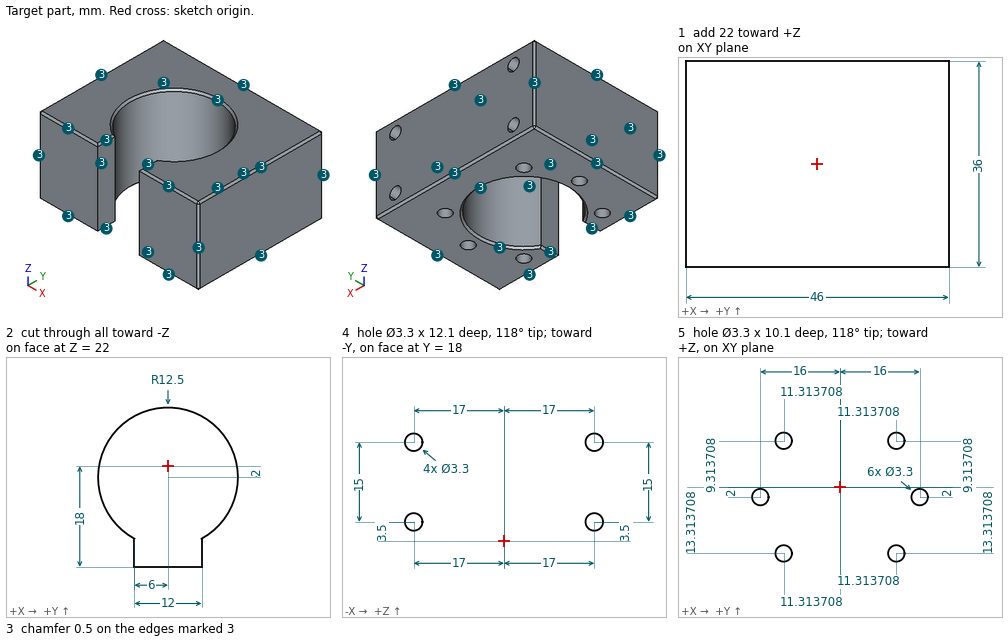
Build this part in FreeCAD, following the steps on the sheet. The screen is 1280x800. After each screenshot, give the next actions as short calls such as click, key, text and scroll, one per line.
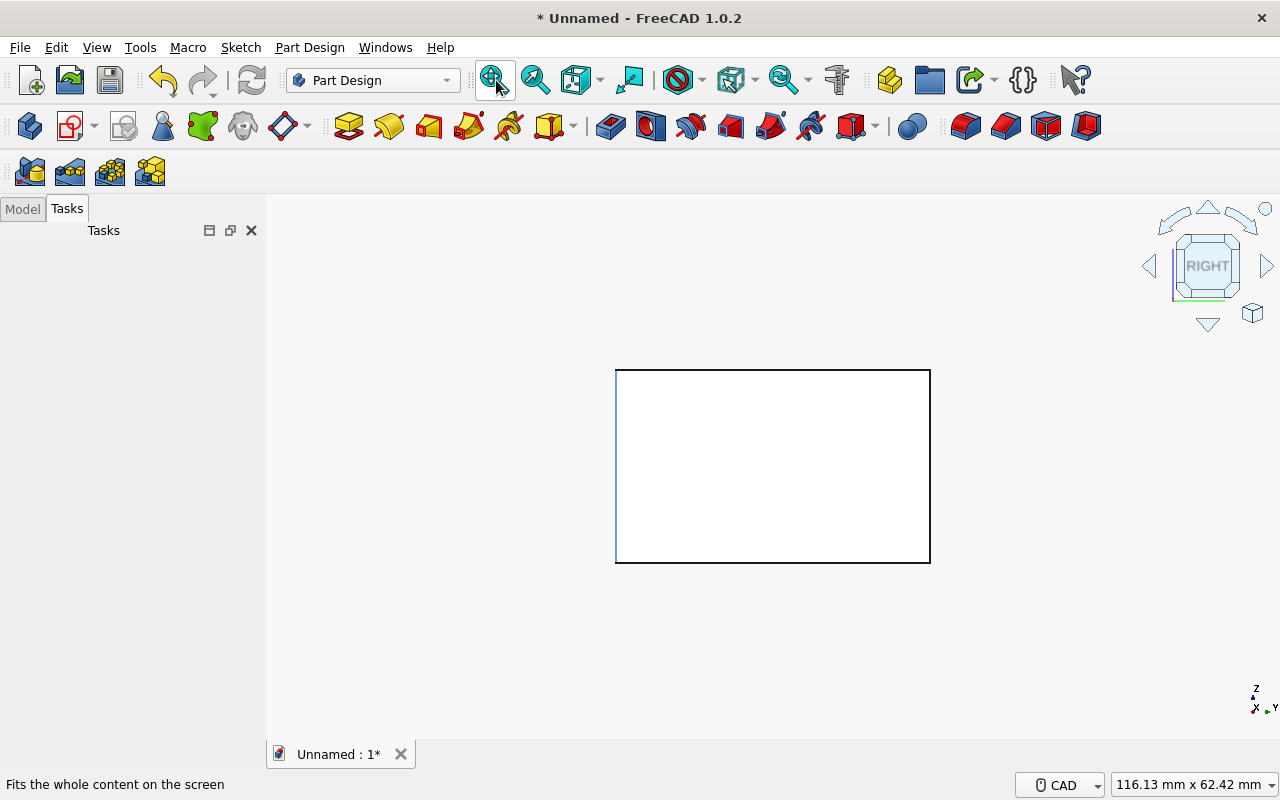
click(930, 465, ctrl)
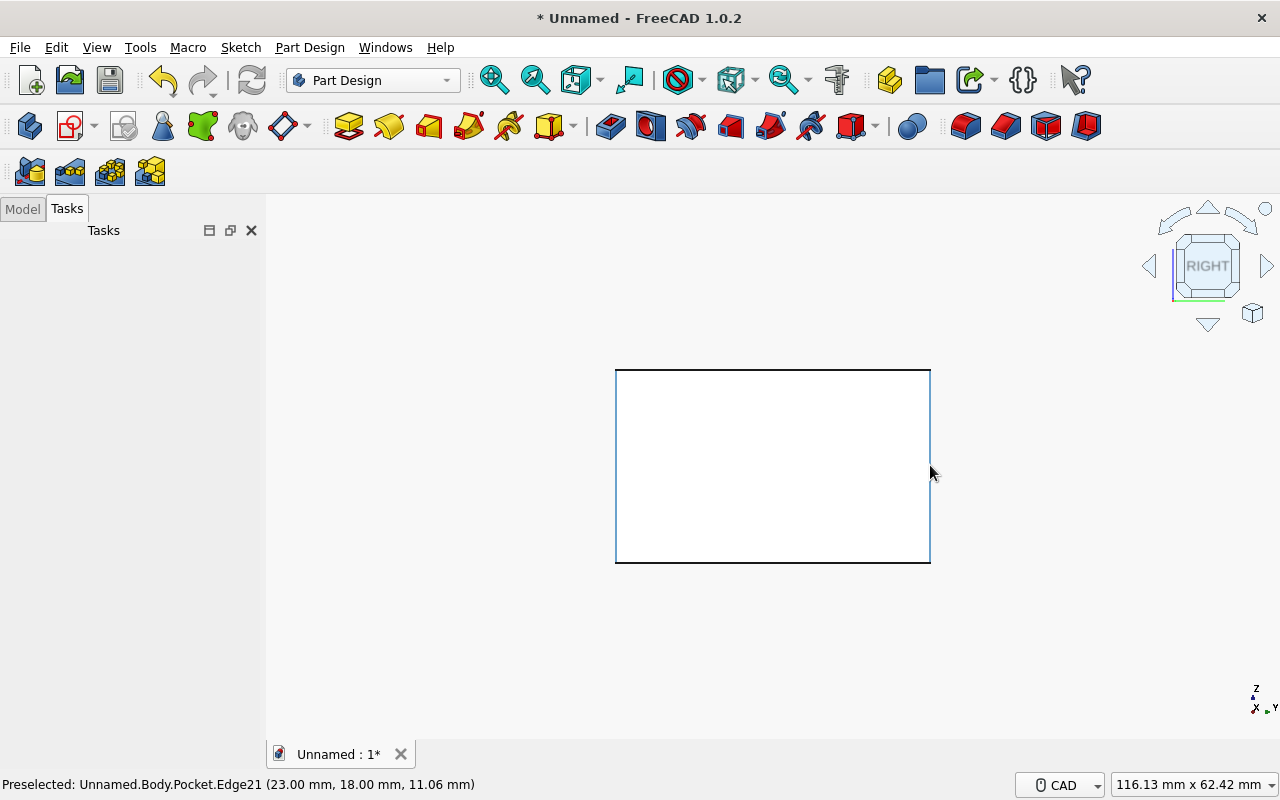
key(5)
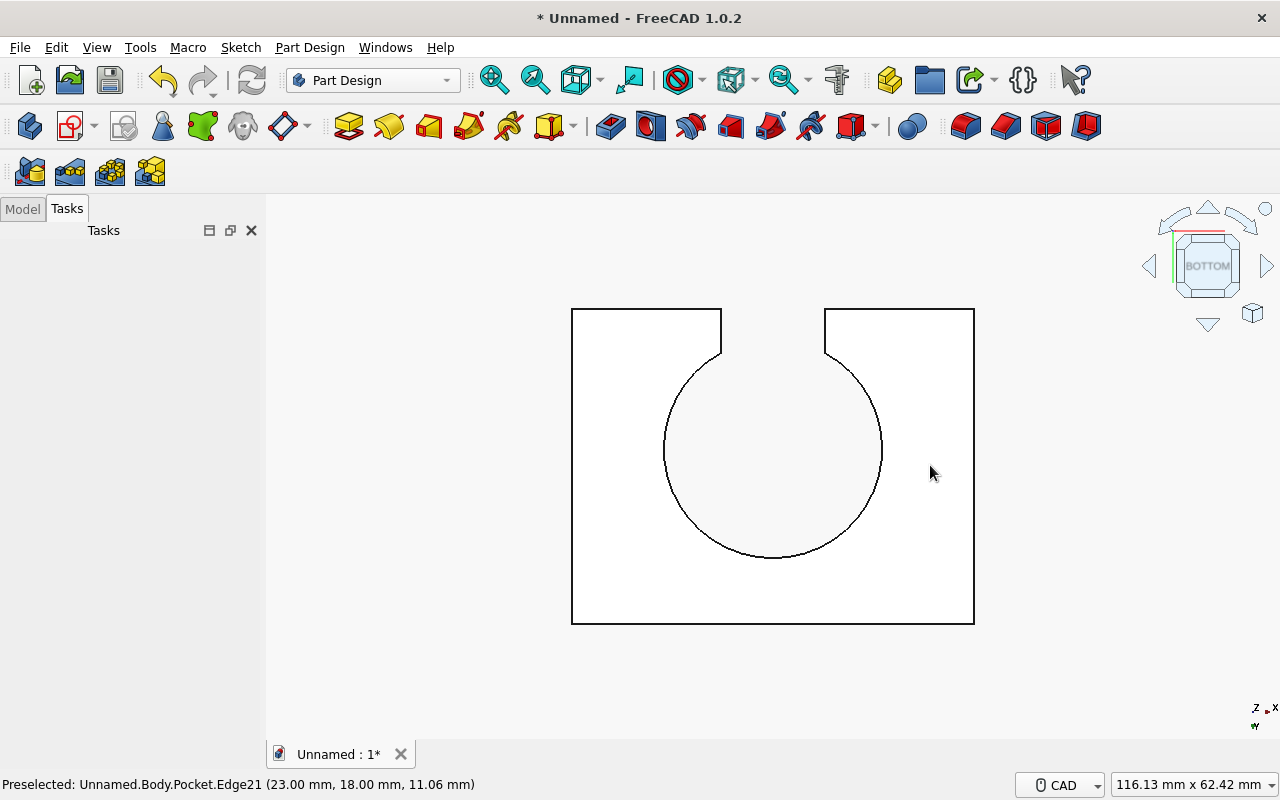
click(888, 555, ctrl)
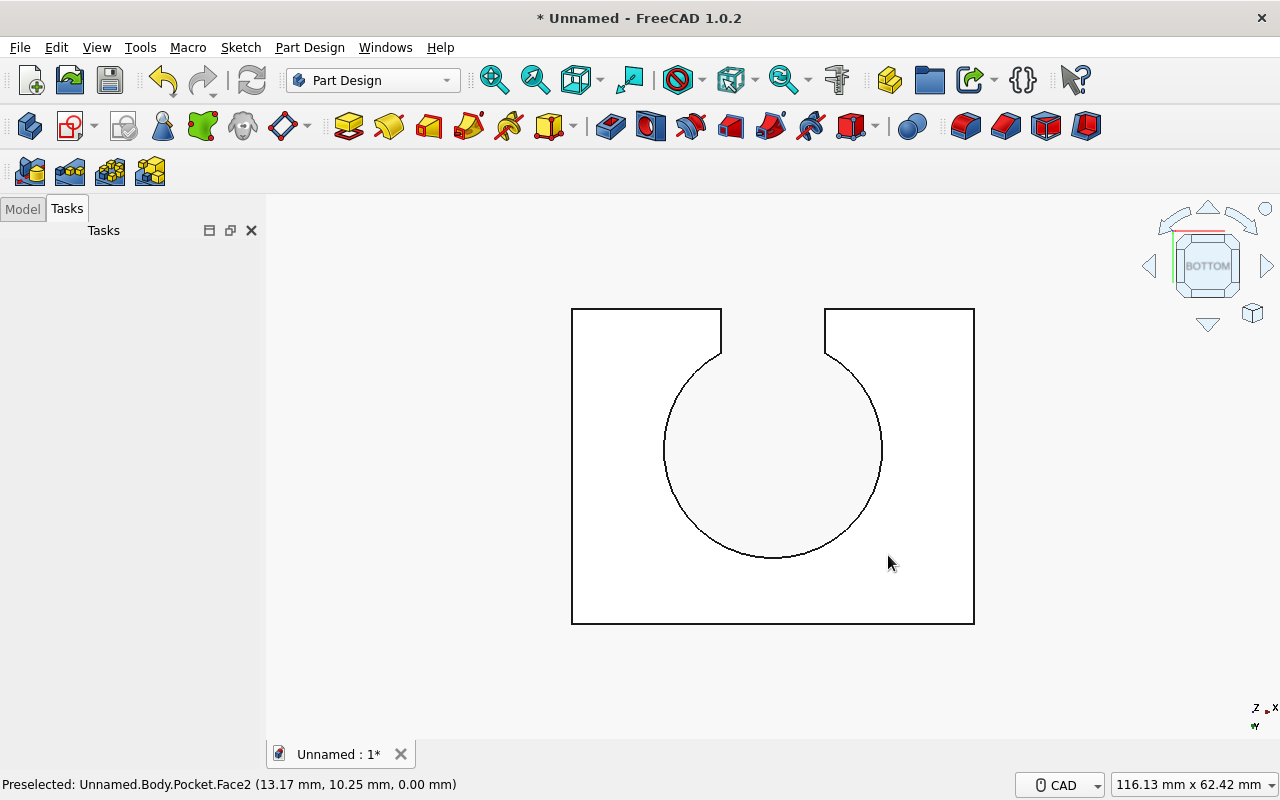
key(4)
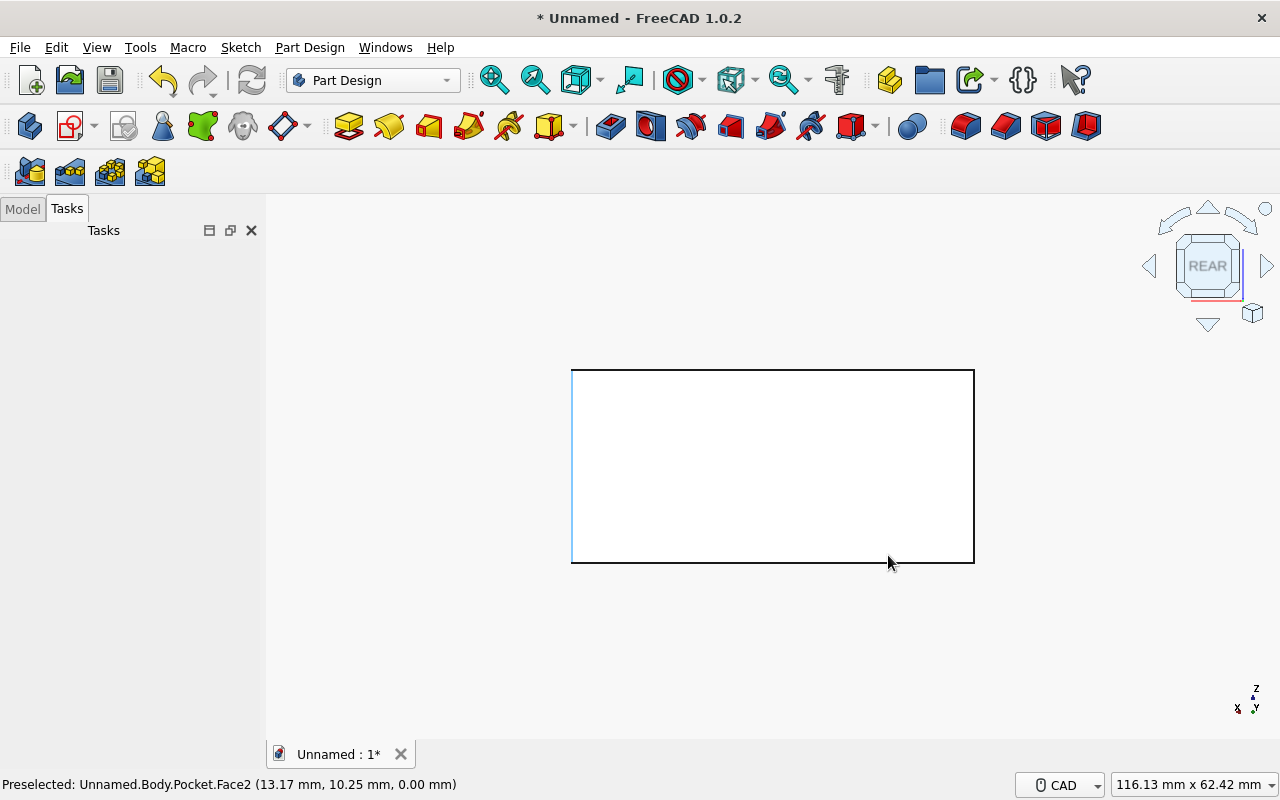
click(496, 80)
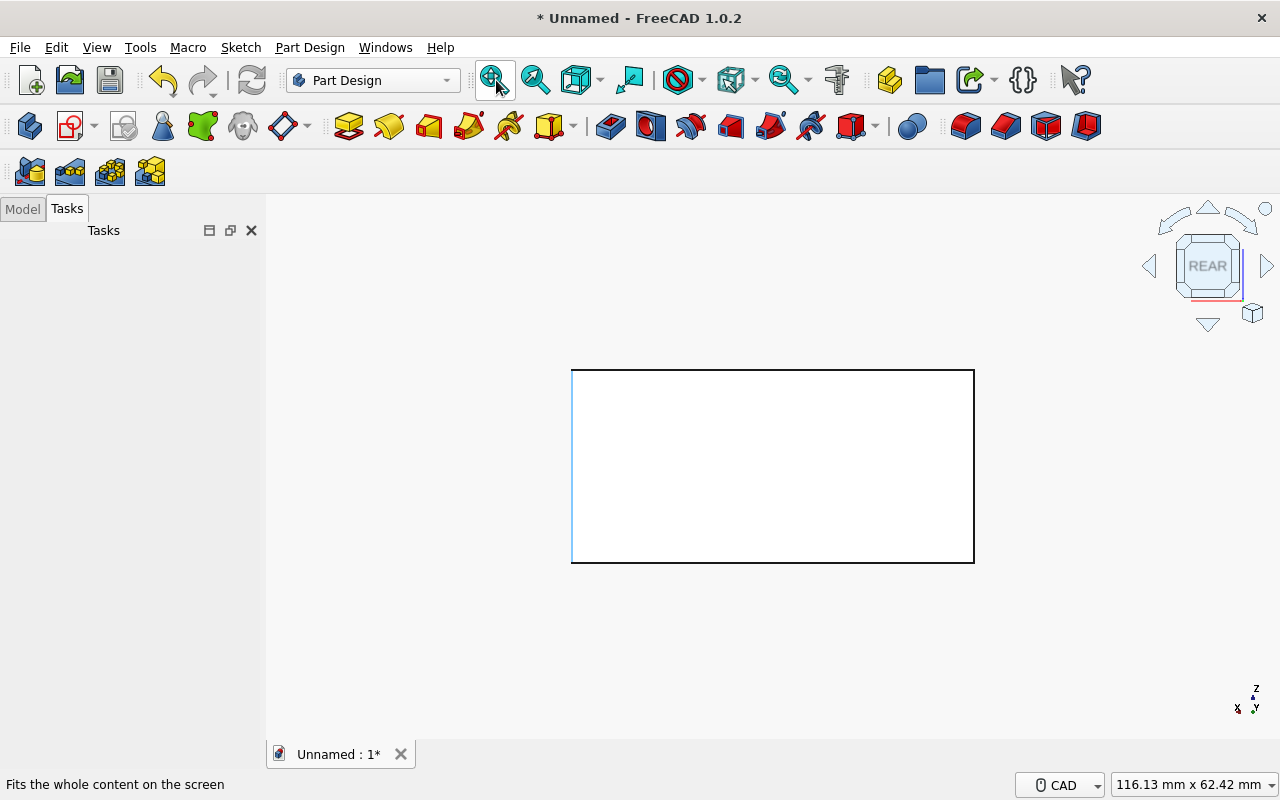
click(974, 466, ctrl)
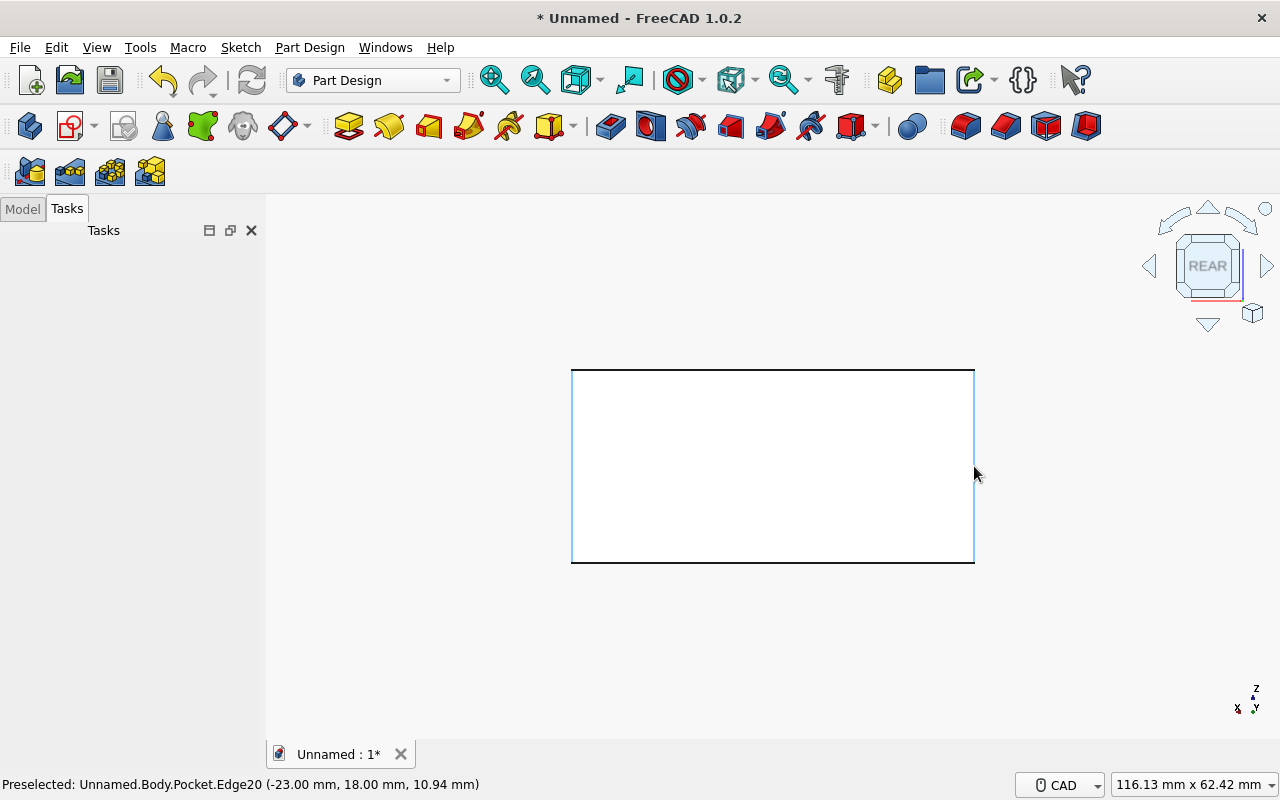
click(1006, 126)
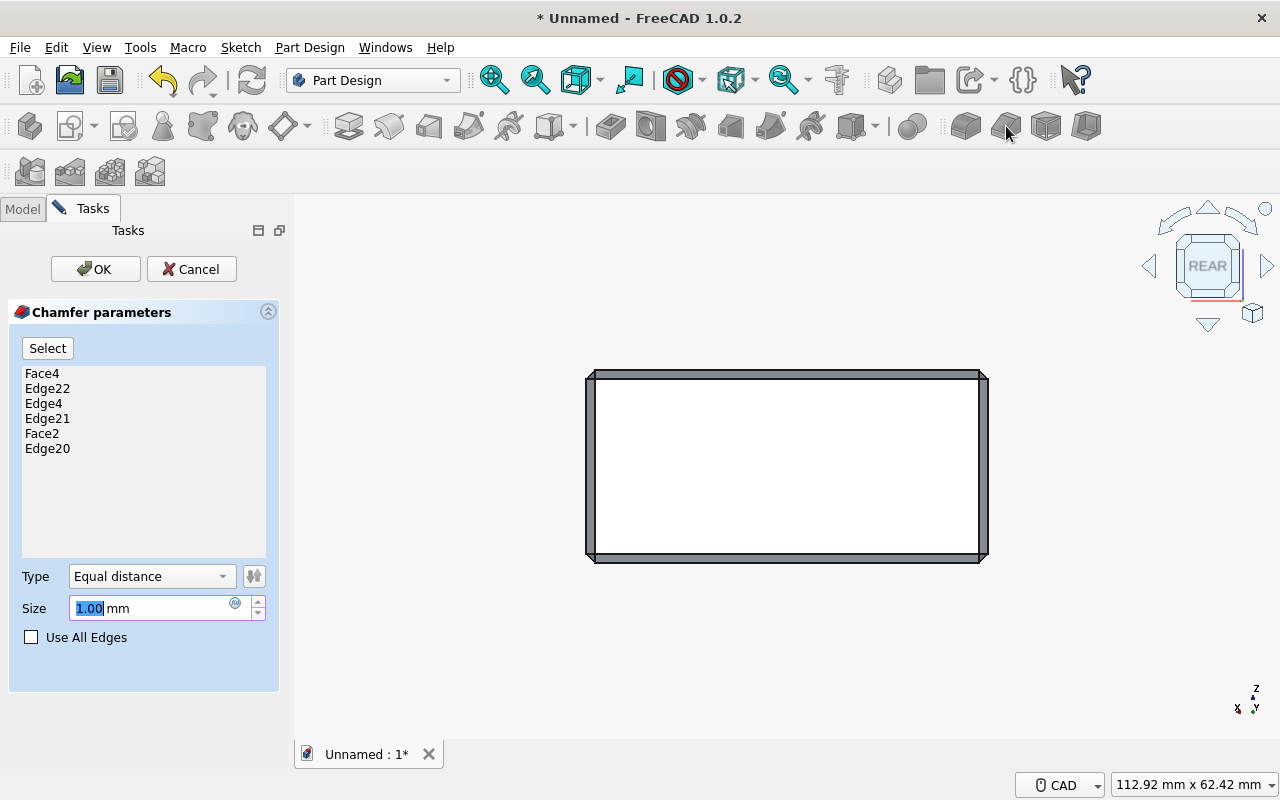
text(0.5)
key(Tab)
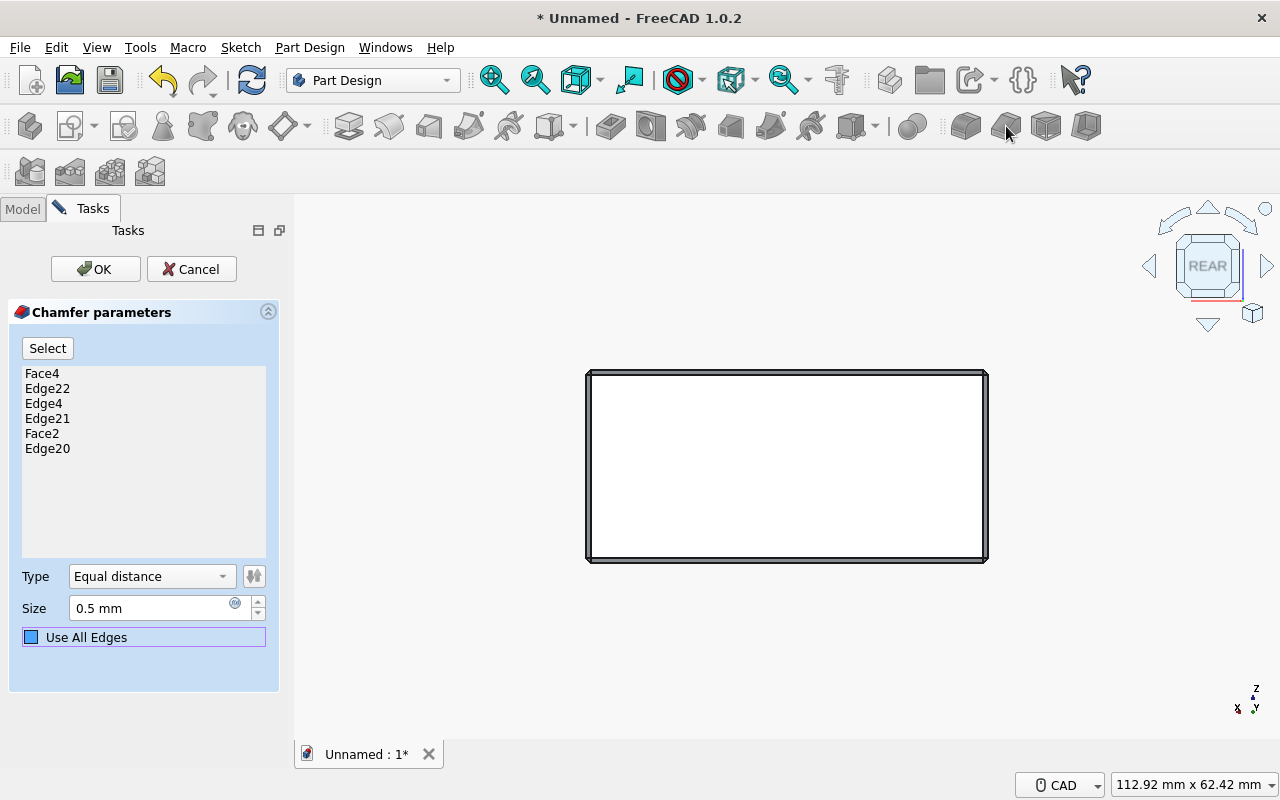
click(96, 269)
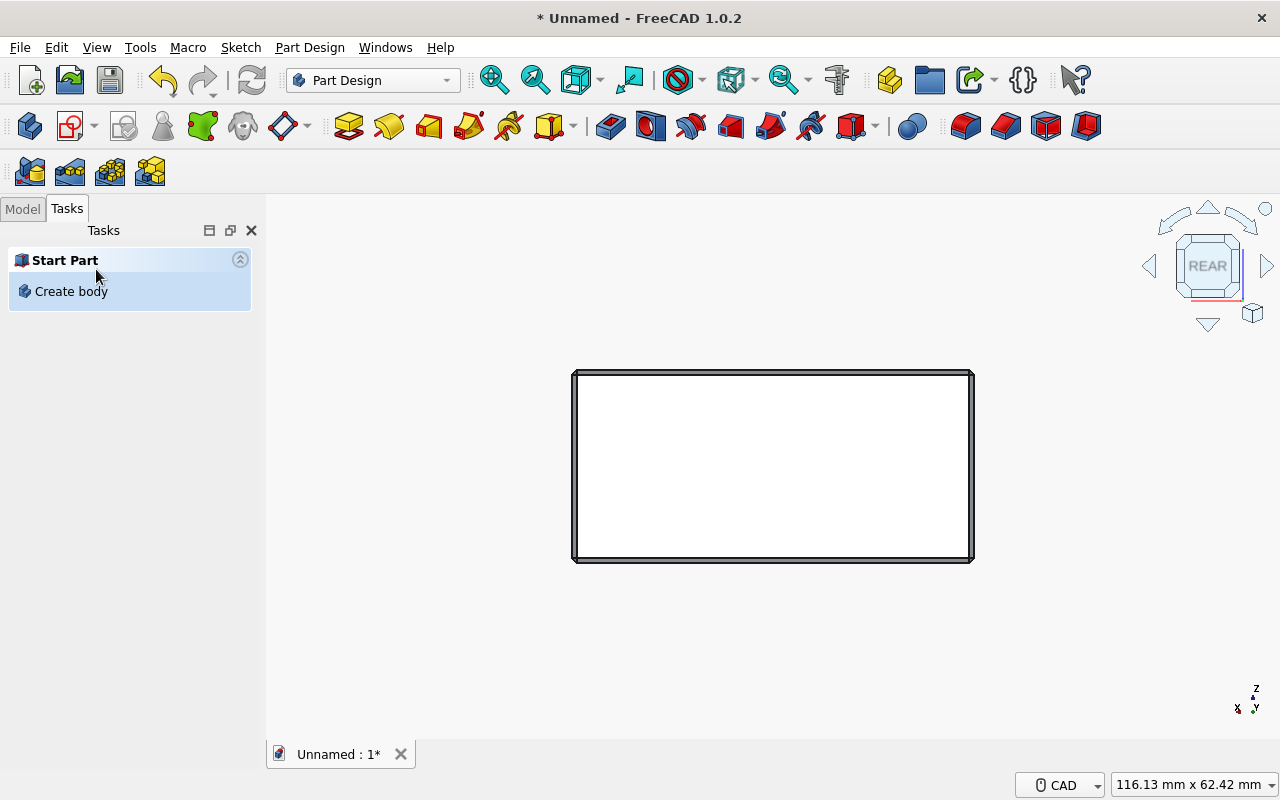
click(496, 80)